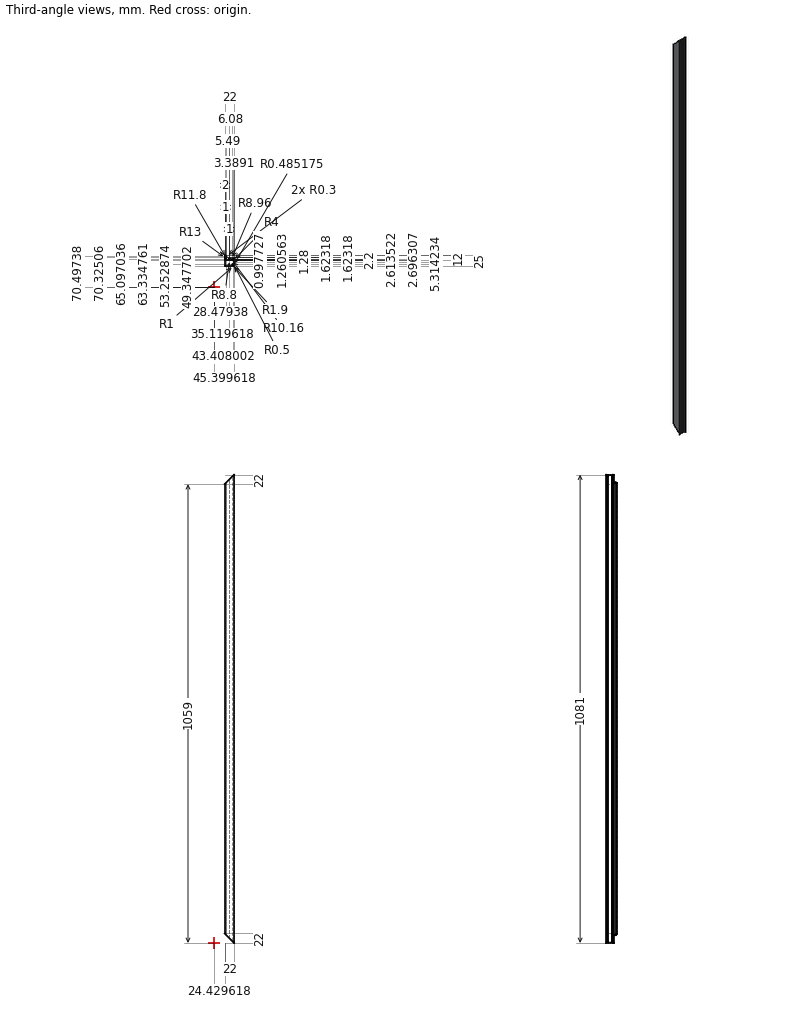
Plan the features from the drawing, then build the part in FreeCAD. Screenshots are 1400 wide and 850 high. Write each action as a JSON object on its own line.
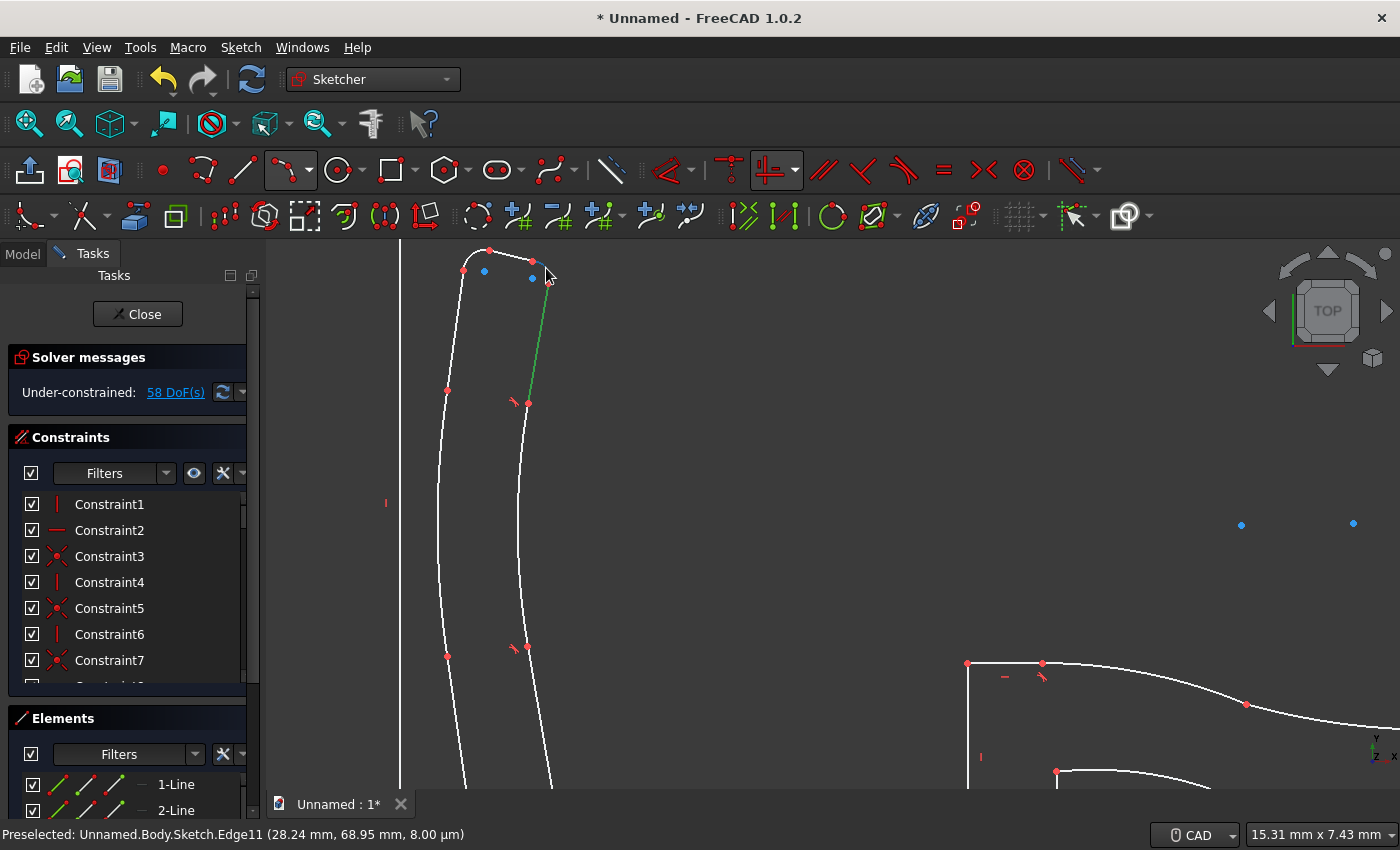
{"action": "left_click", "coordinate": [546, 268]}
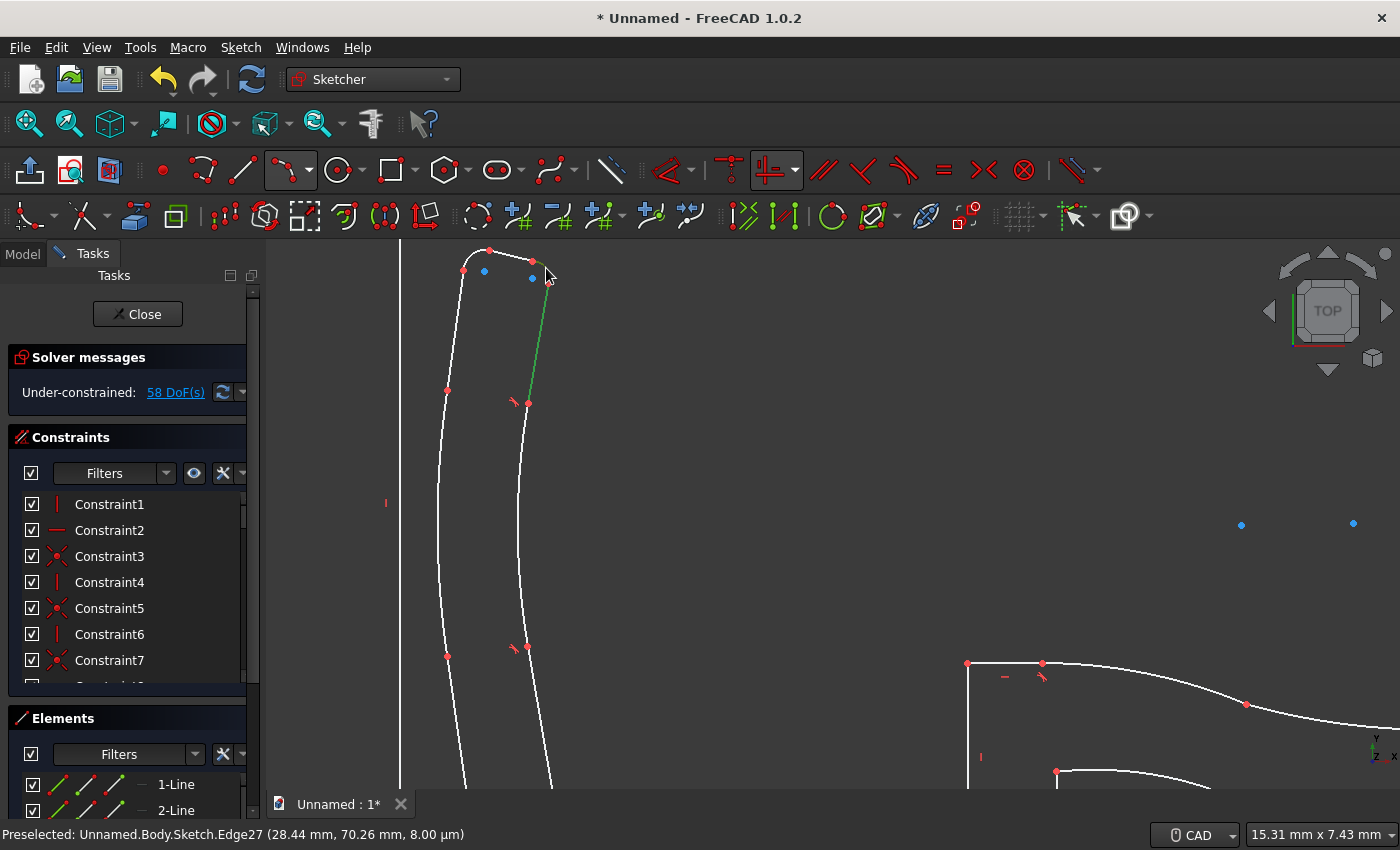
{"action": "left_click", "coordinate": [904, 170]}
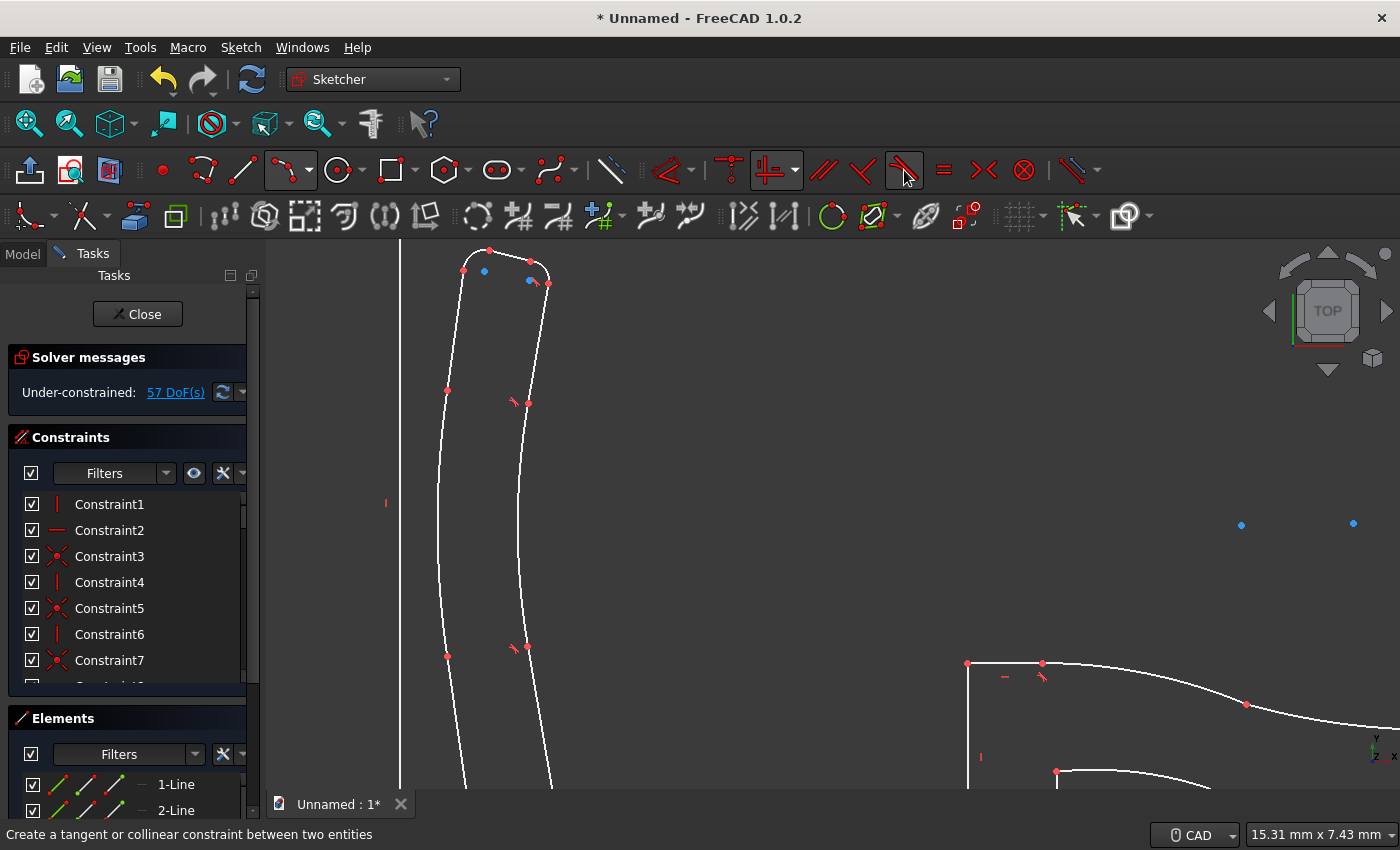
{"action": "scroll", "coordinate": [688, 396], "scroll_direction": "down", "scroll_amount": 8}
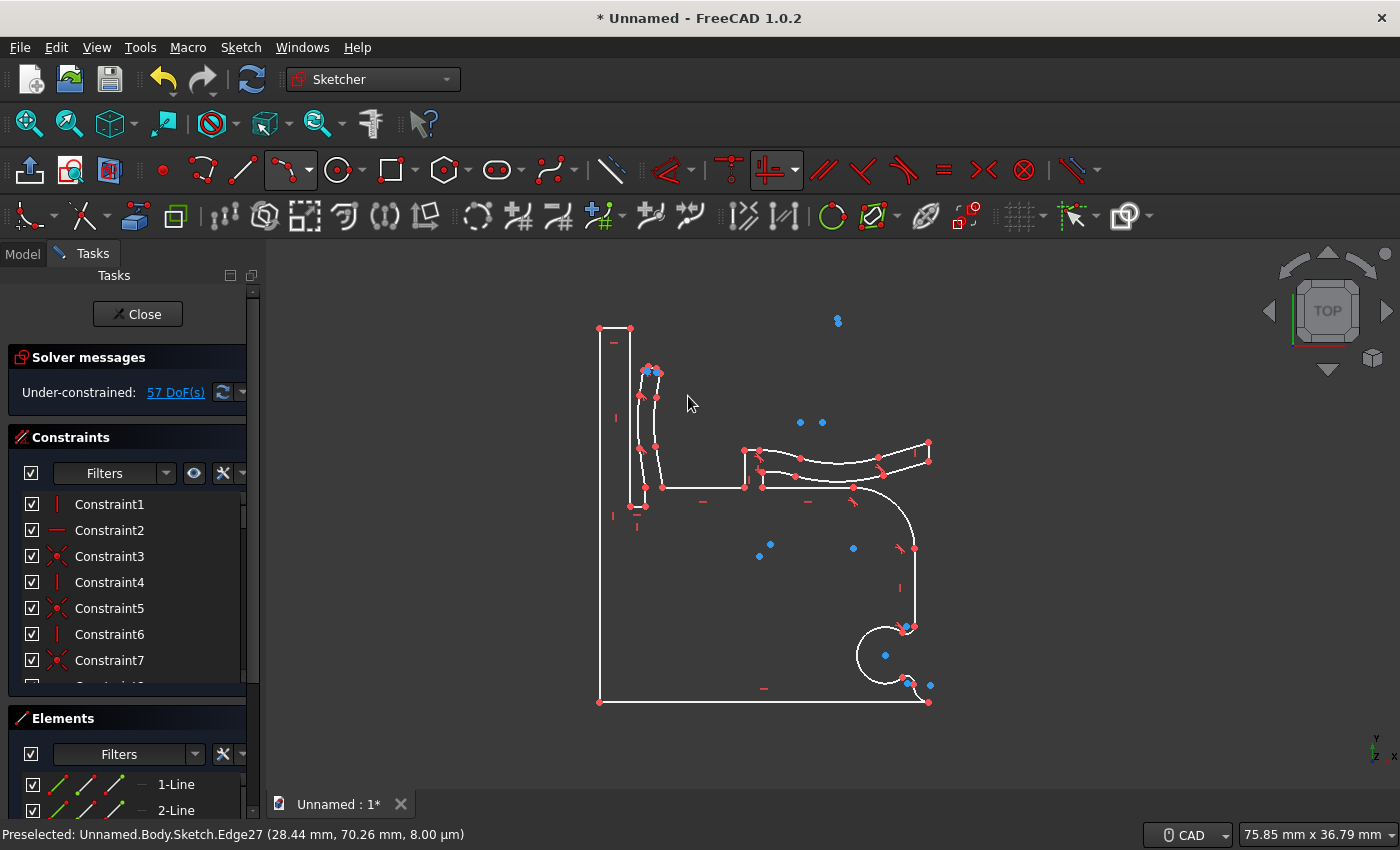
{"action": "scroll", "coordinate": [654, 368], "scroll_direction": "up", "scroll_amount": 9}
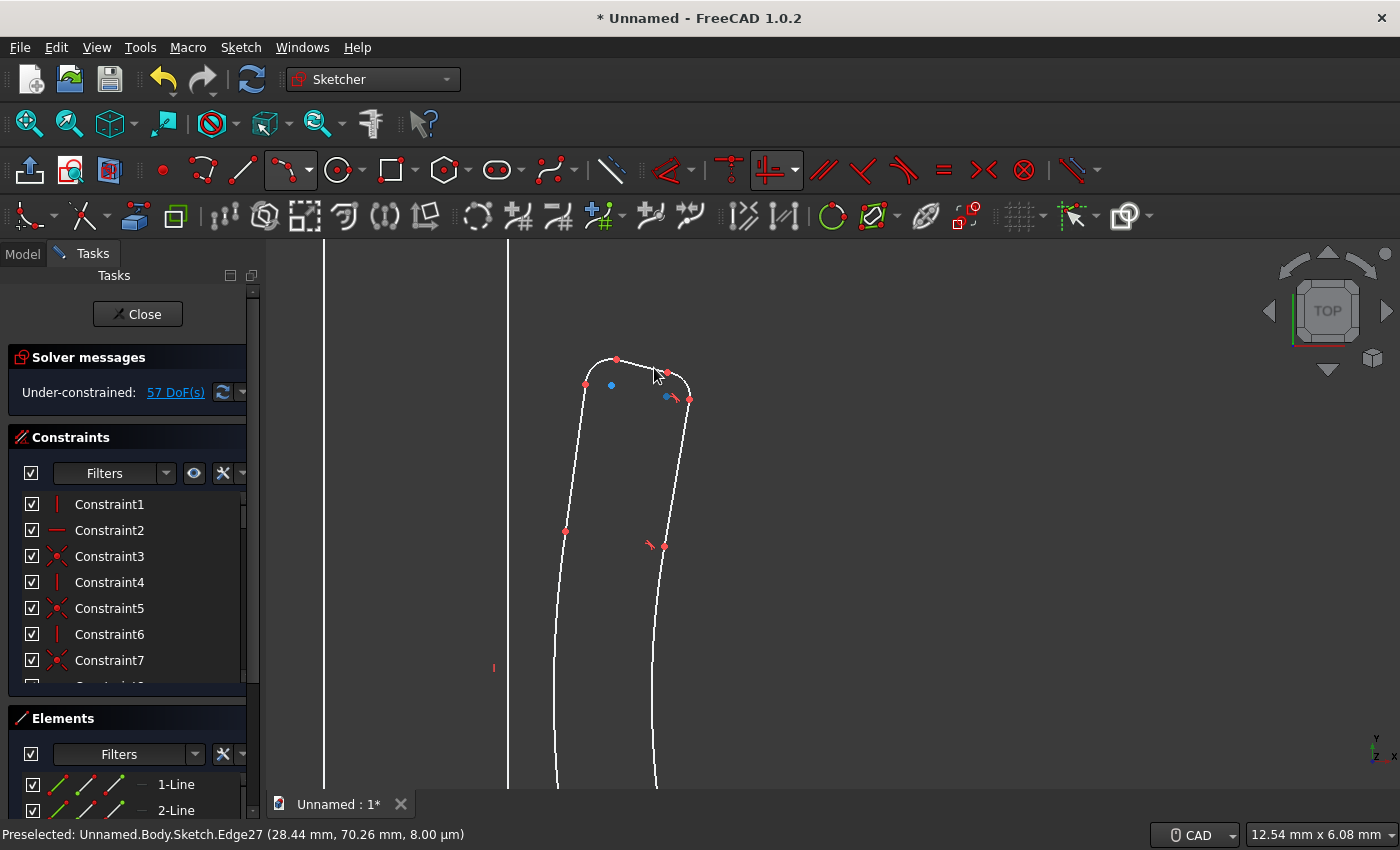
{"action": "left_click", "coordinate": [652, 369]}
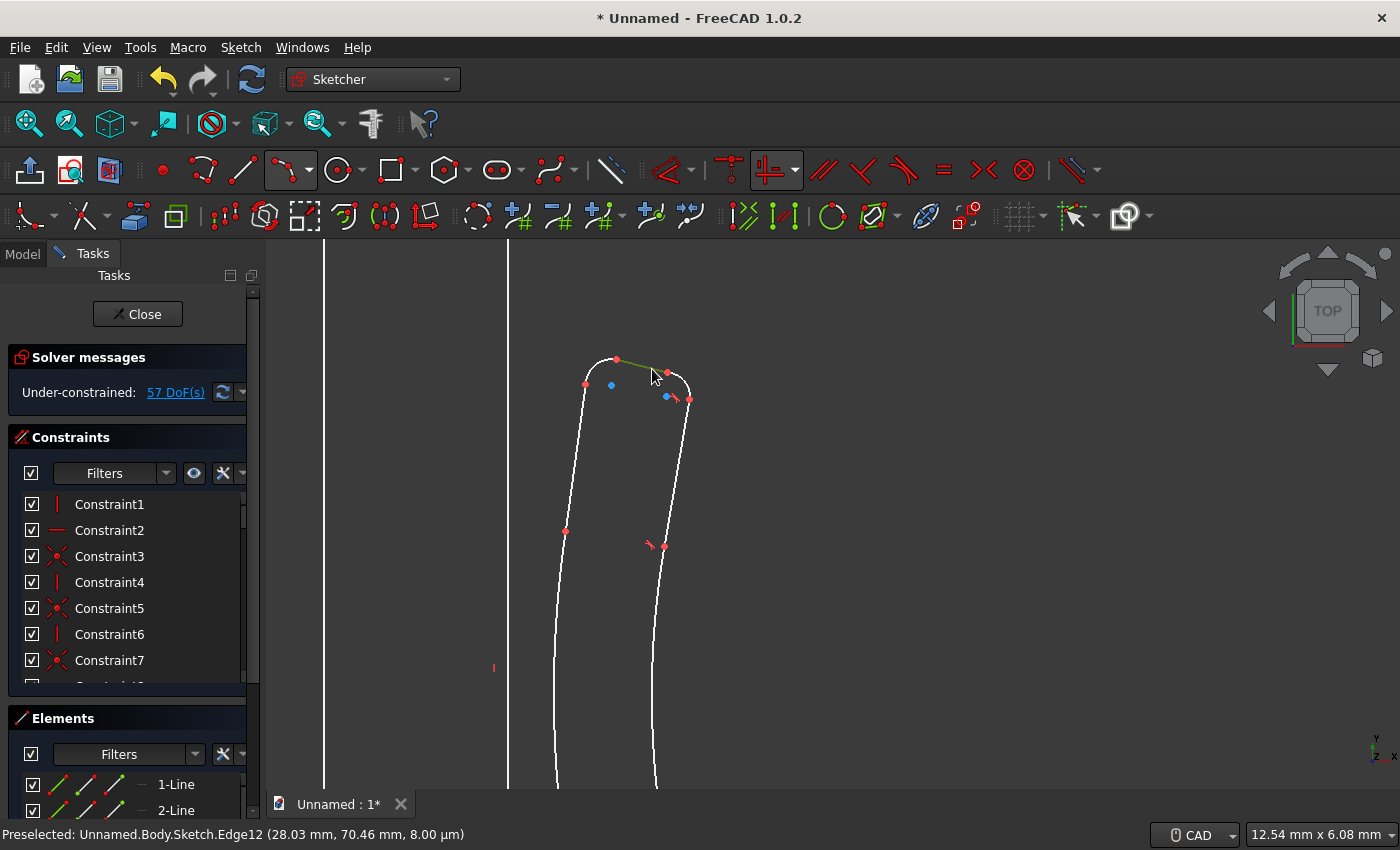
{"action": "left_click", "coordinate": [688, 388]}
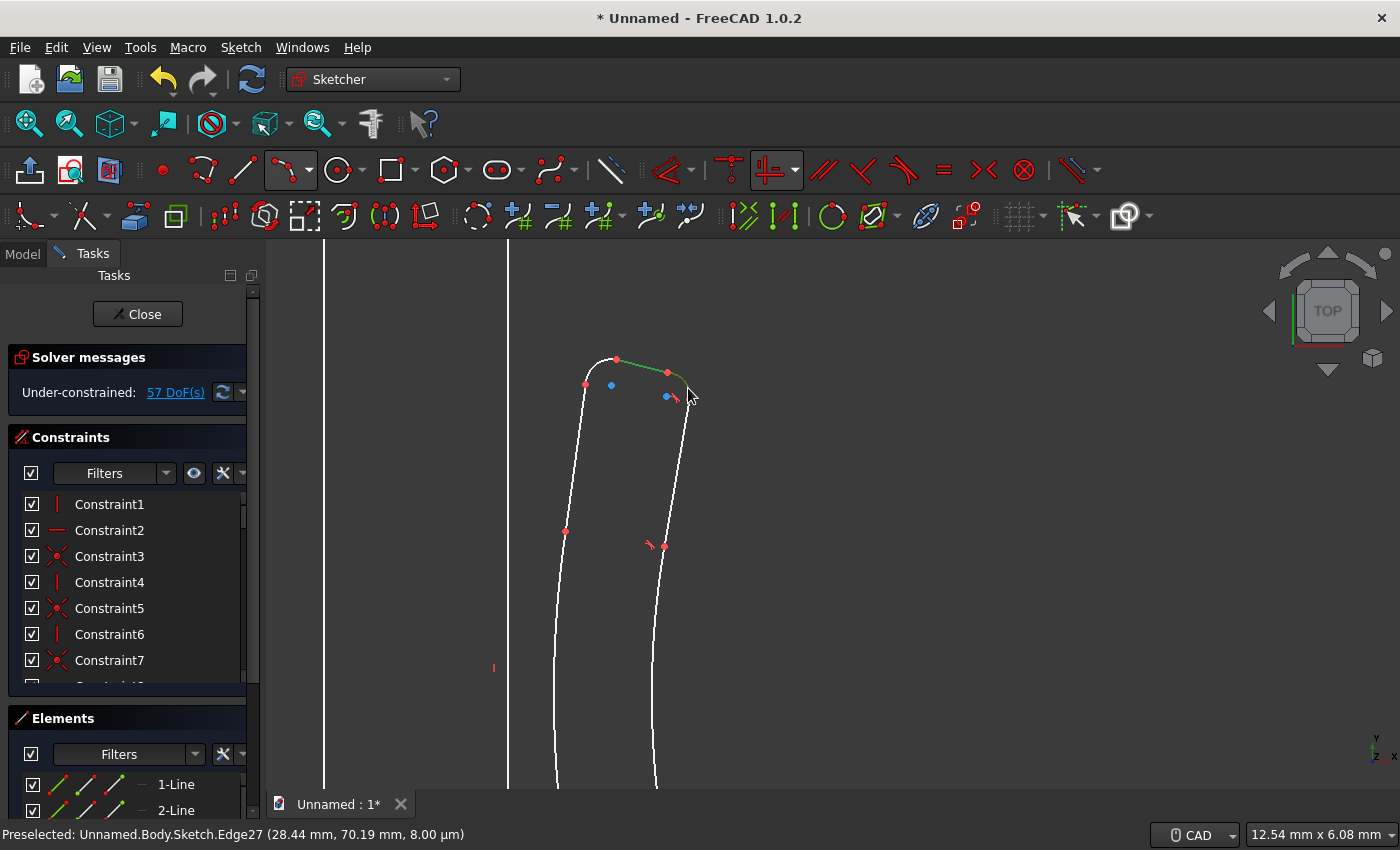
{"action": "left_click", "coordinate": [904, 170]}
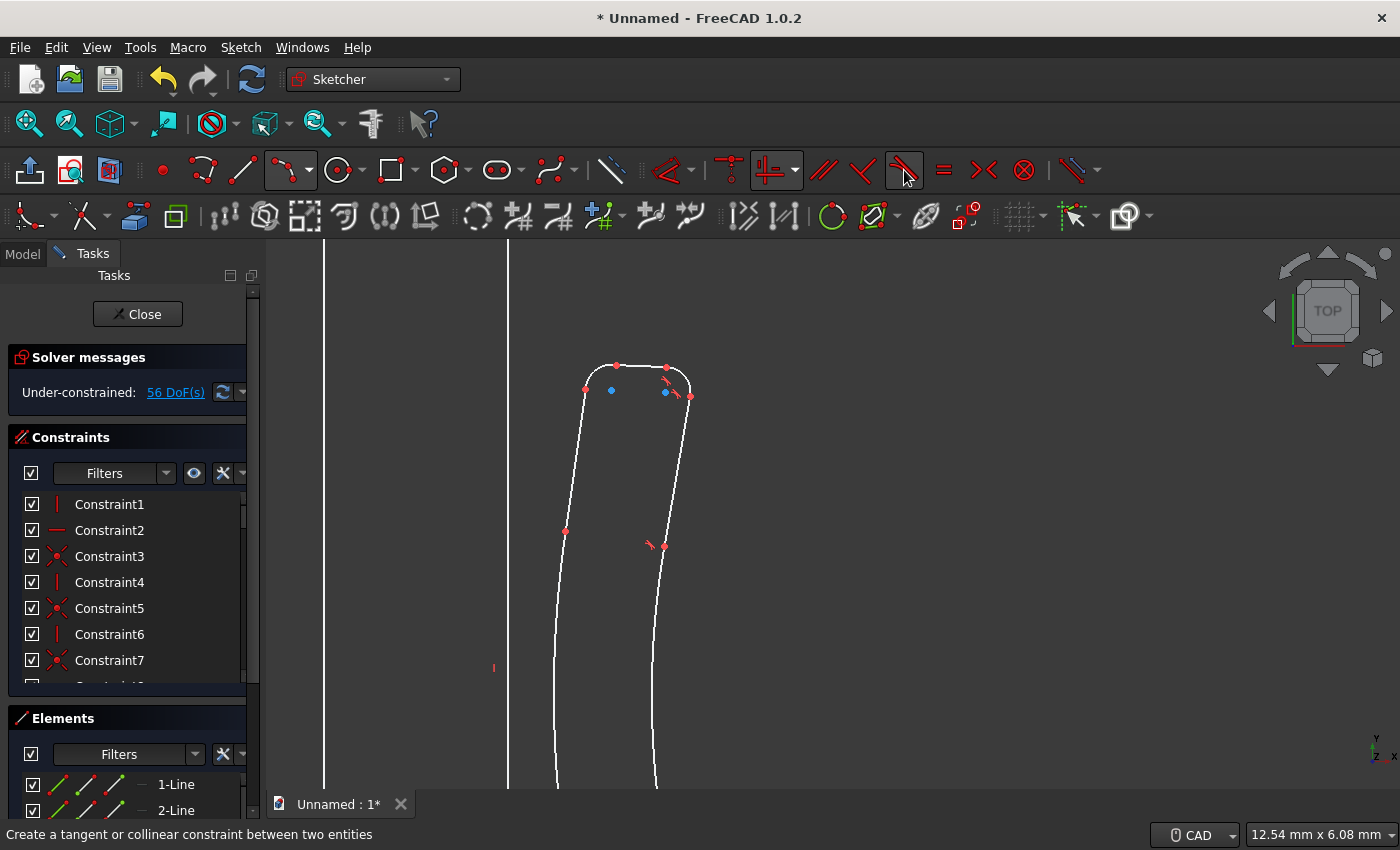
{"action": "left_click", "coordinate": [652, 367]}